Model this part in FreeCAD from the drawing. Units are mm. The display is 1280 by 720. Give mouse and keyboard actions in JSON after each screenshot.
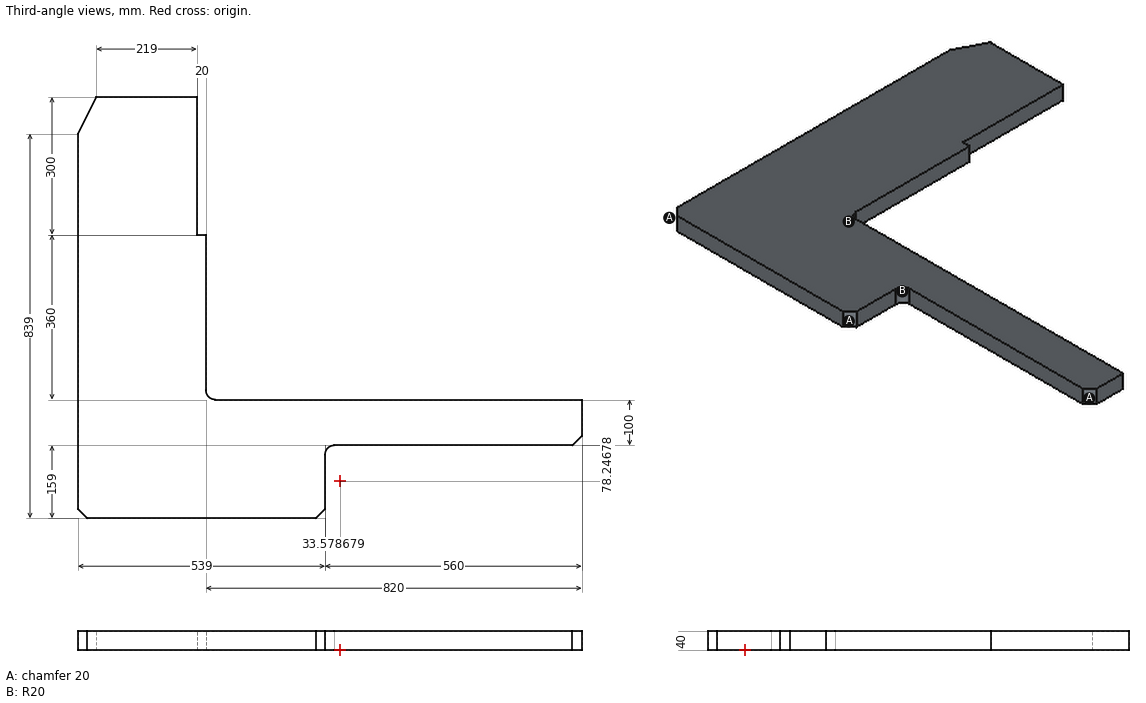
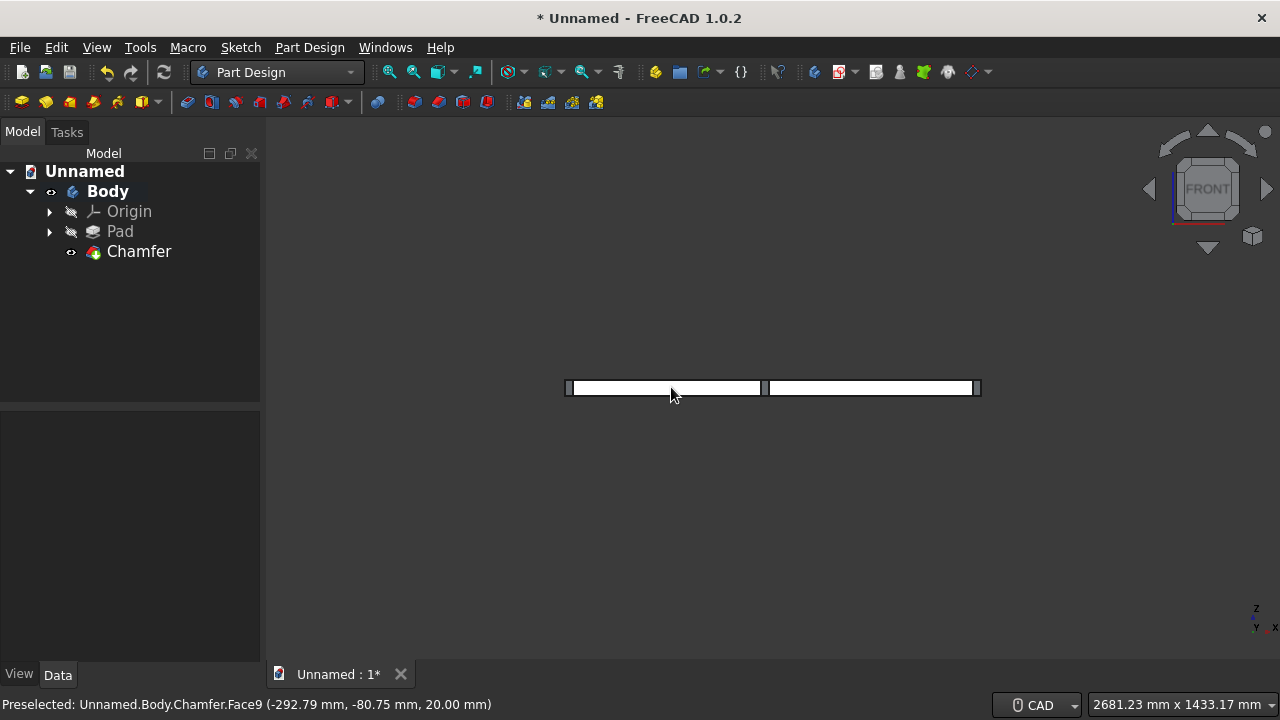
{"action": "key", "text": "3"}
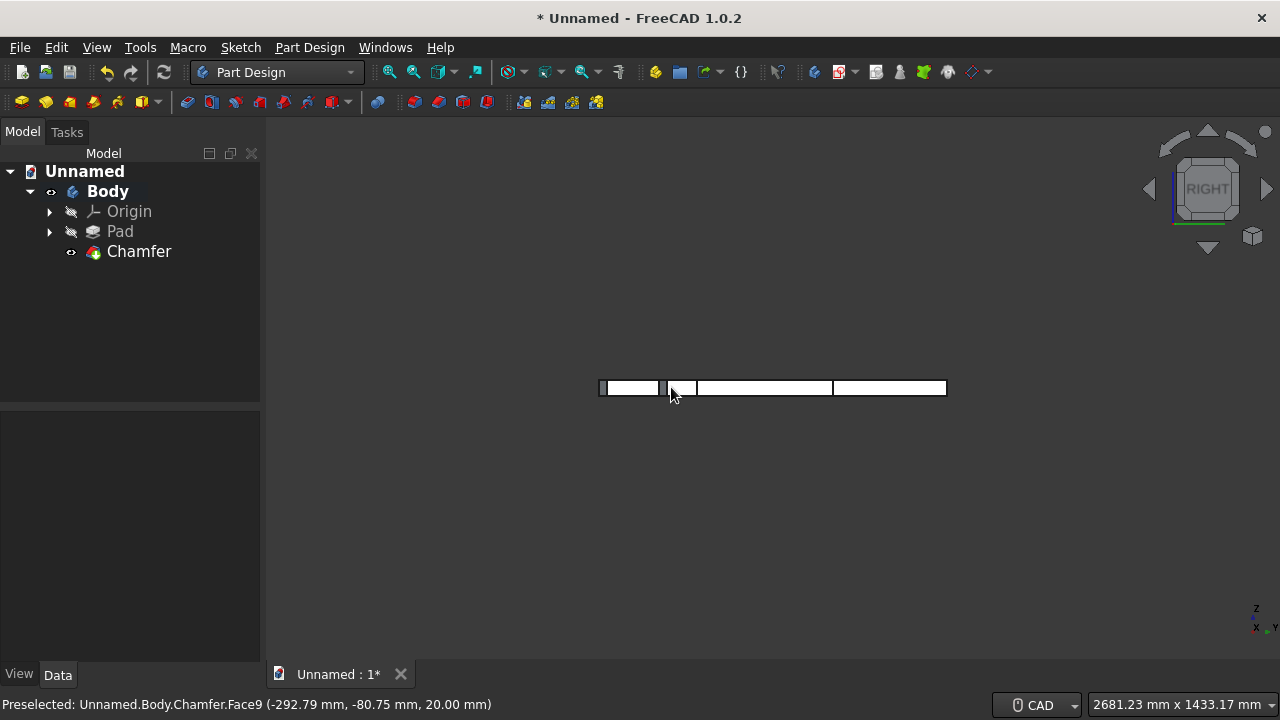
{"action": "key", "text": "v f"}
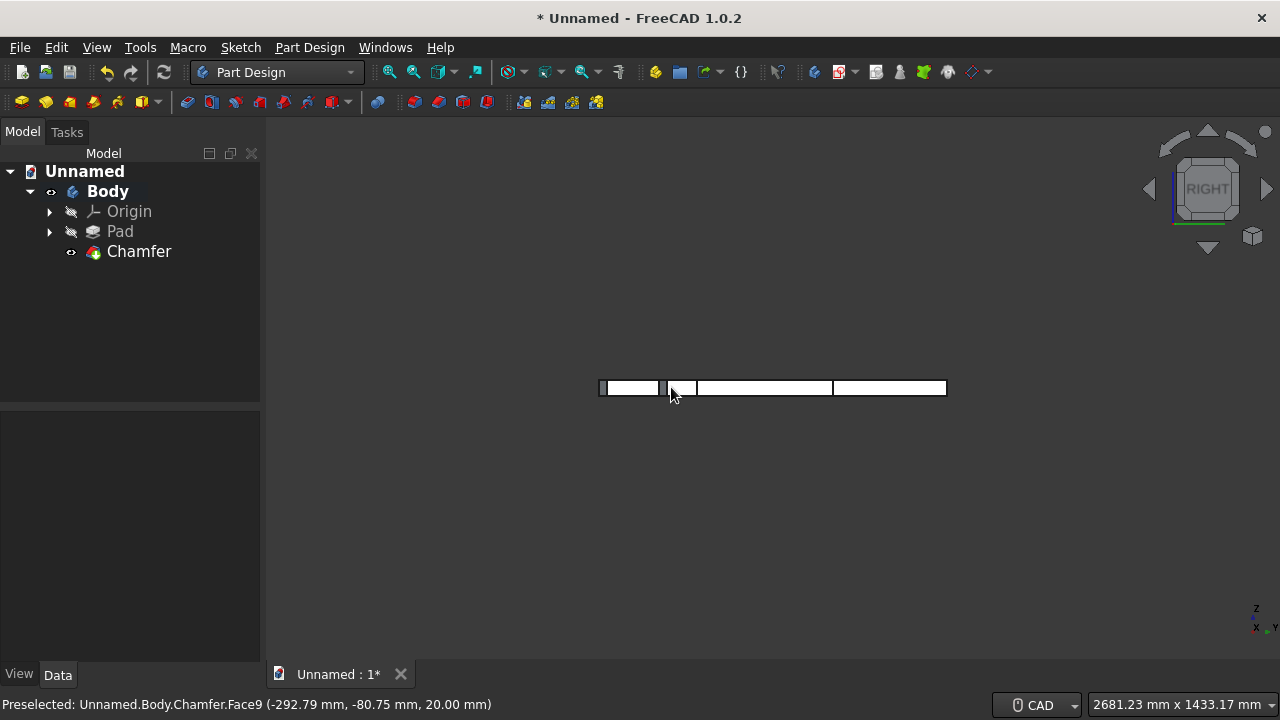
{"action": "scroll", "coordinate": [697, 387], "scroll_direction": "up", "scroll_amount": 5}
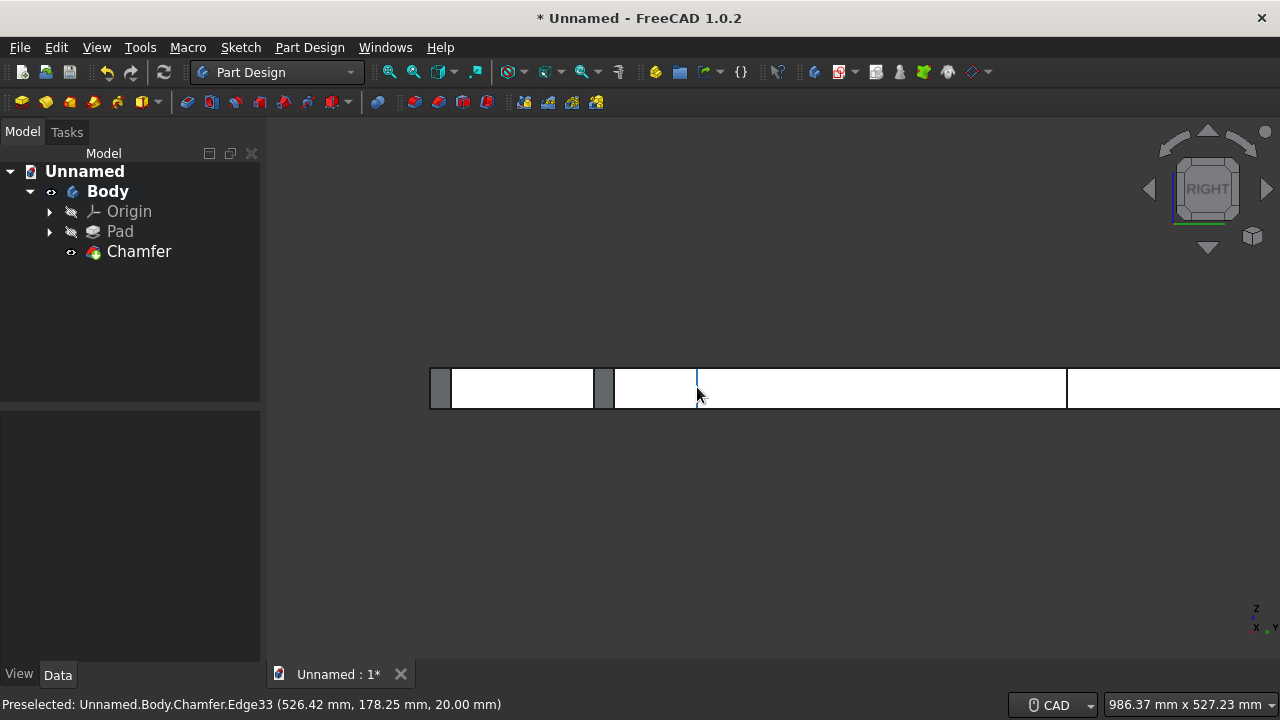
{"action": "key", "text": "v f"}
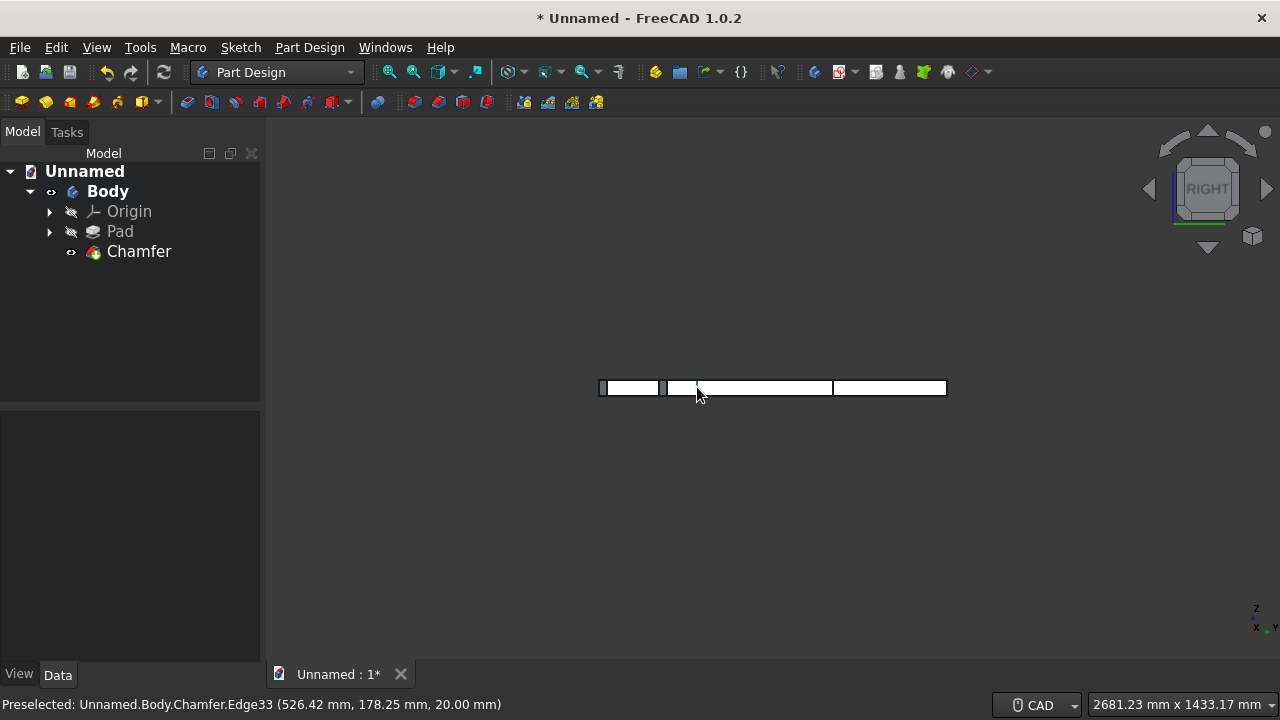
{"action": "key", "text": "5"}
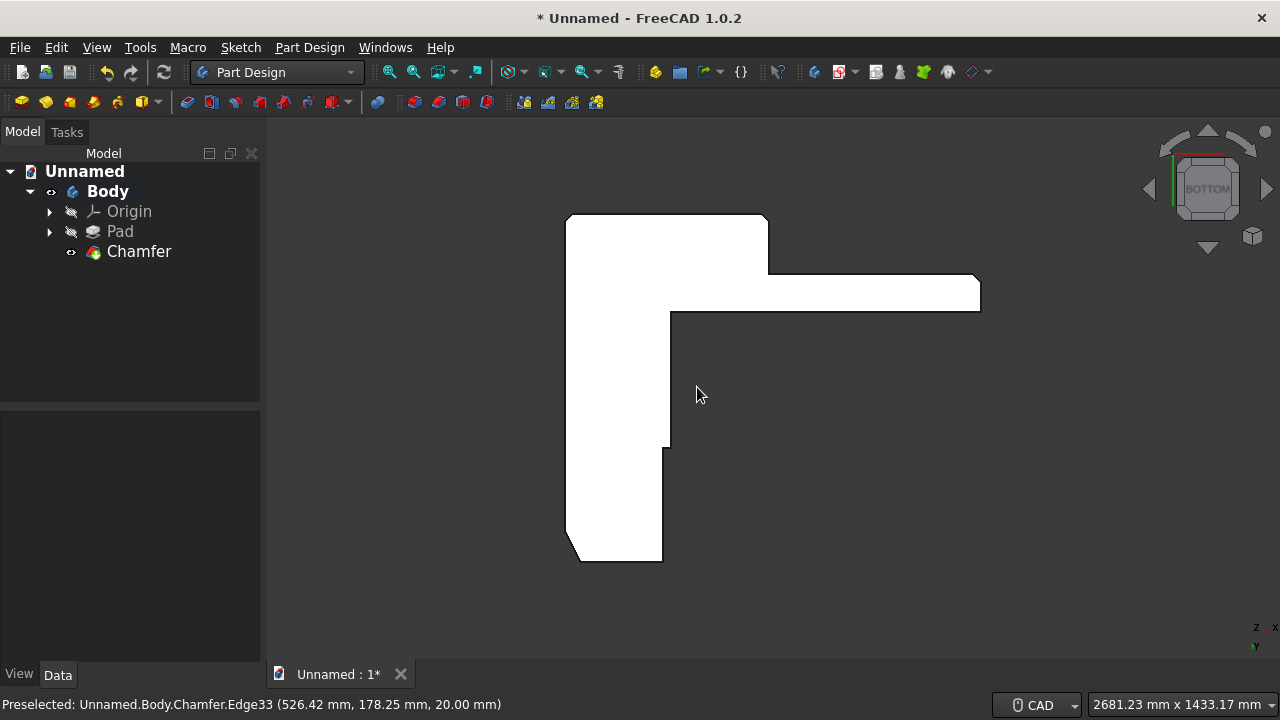
{"action": "scroll", "coordinate": [671, 311], "scroll_direction": "up", "scroll_amount": 5}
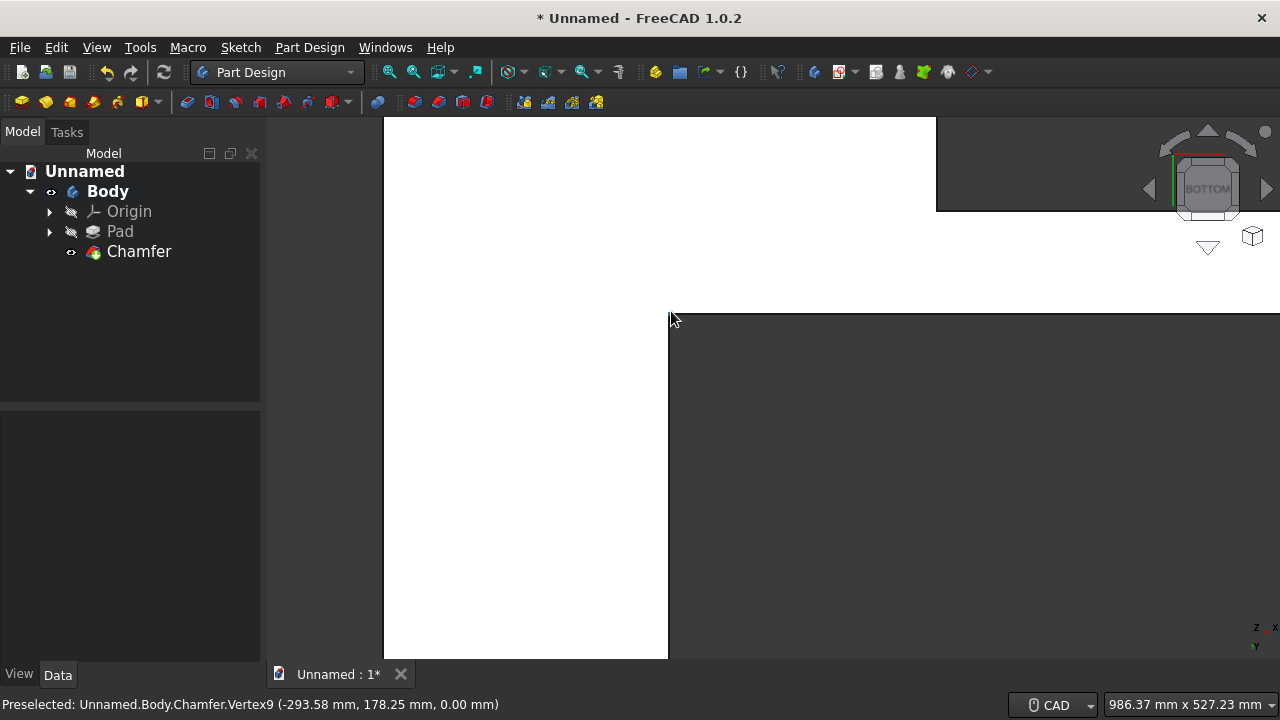
{"action": "key", "text": "v f"}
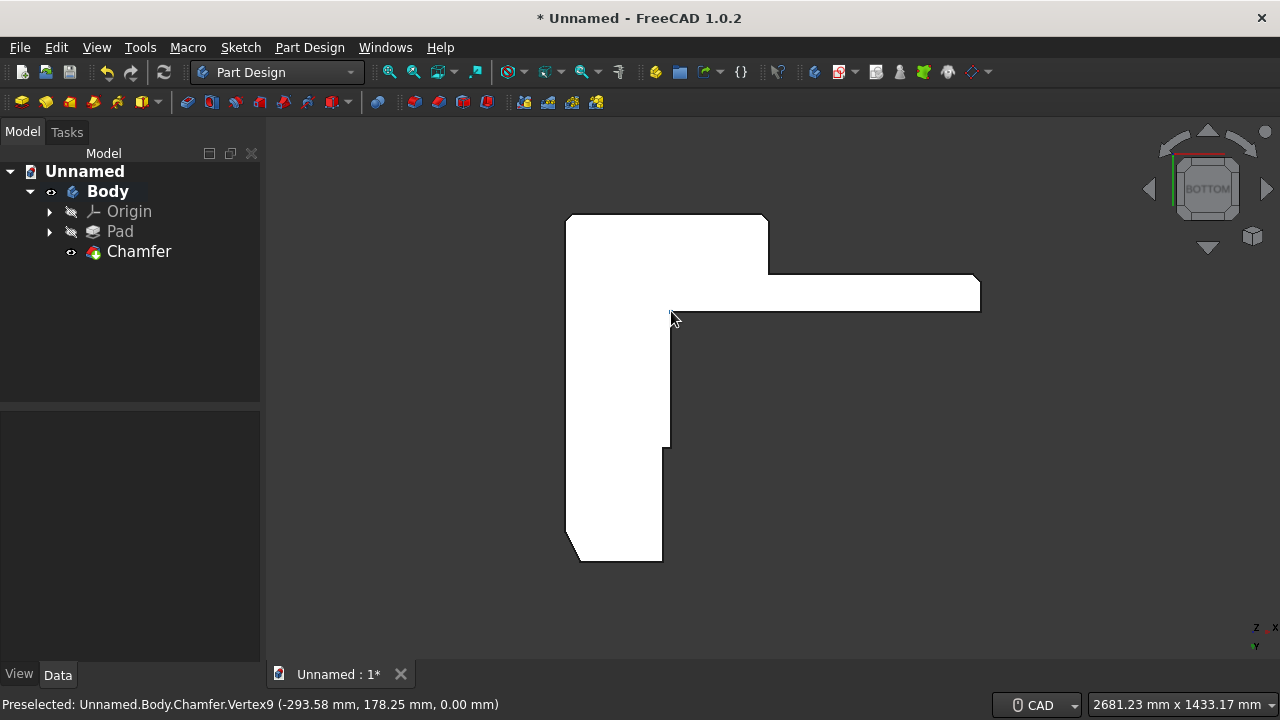
{"action": "key", "text": "4"}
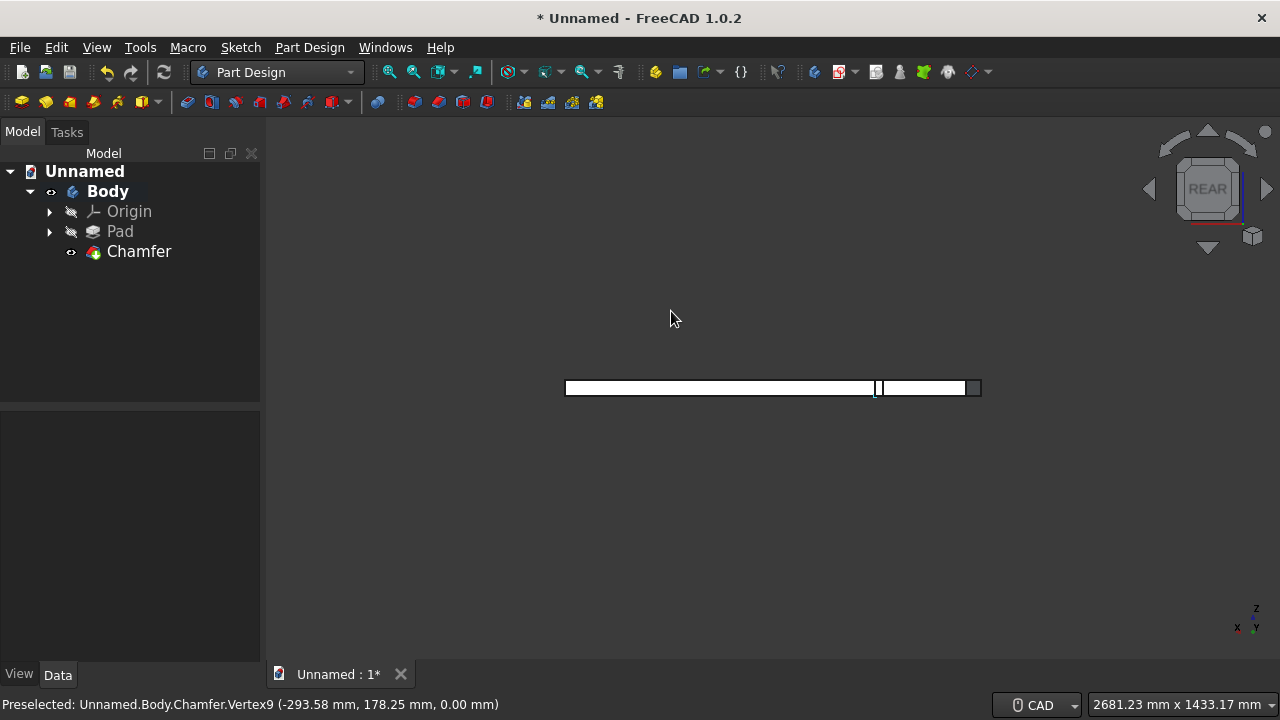
{"action": "key", "text": "v f"}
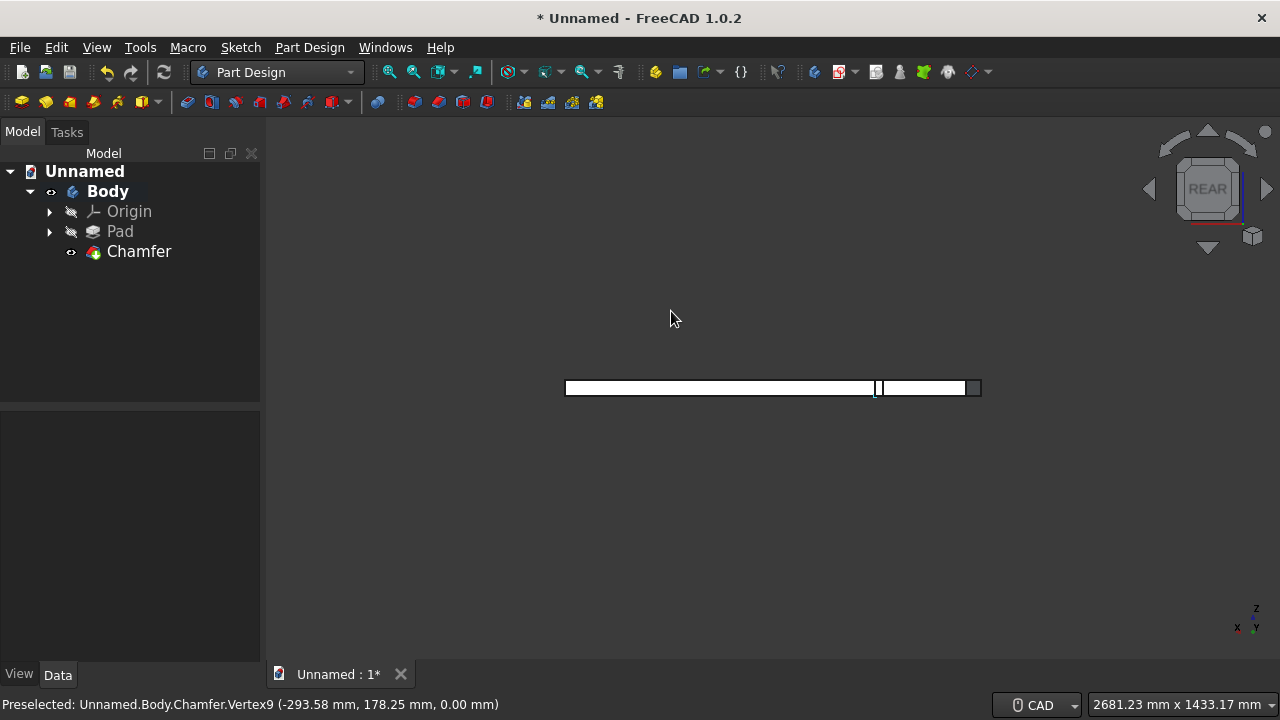
{"action": "scroll", "coordinate": [875, 387], "scroll_direction": "up", "scroll_amount": 5}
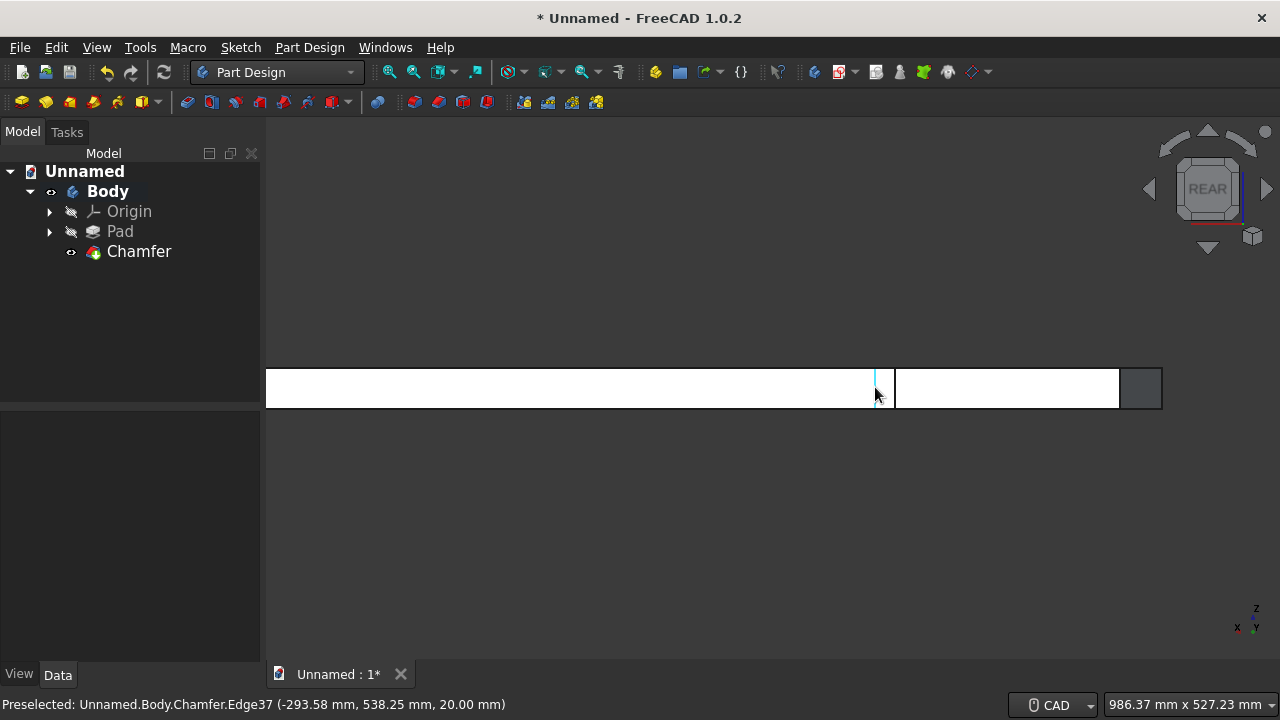
{"action": "key", "text": "v f"}